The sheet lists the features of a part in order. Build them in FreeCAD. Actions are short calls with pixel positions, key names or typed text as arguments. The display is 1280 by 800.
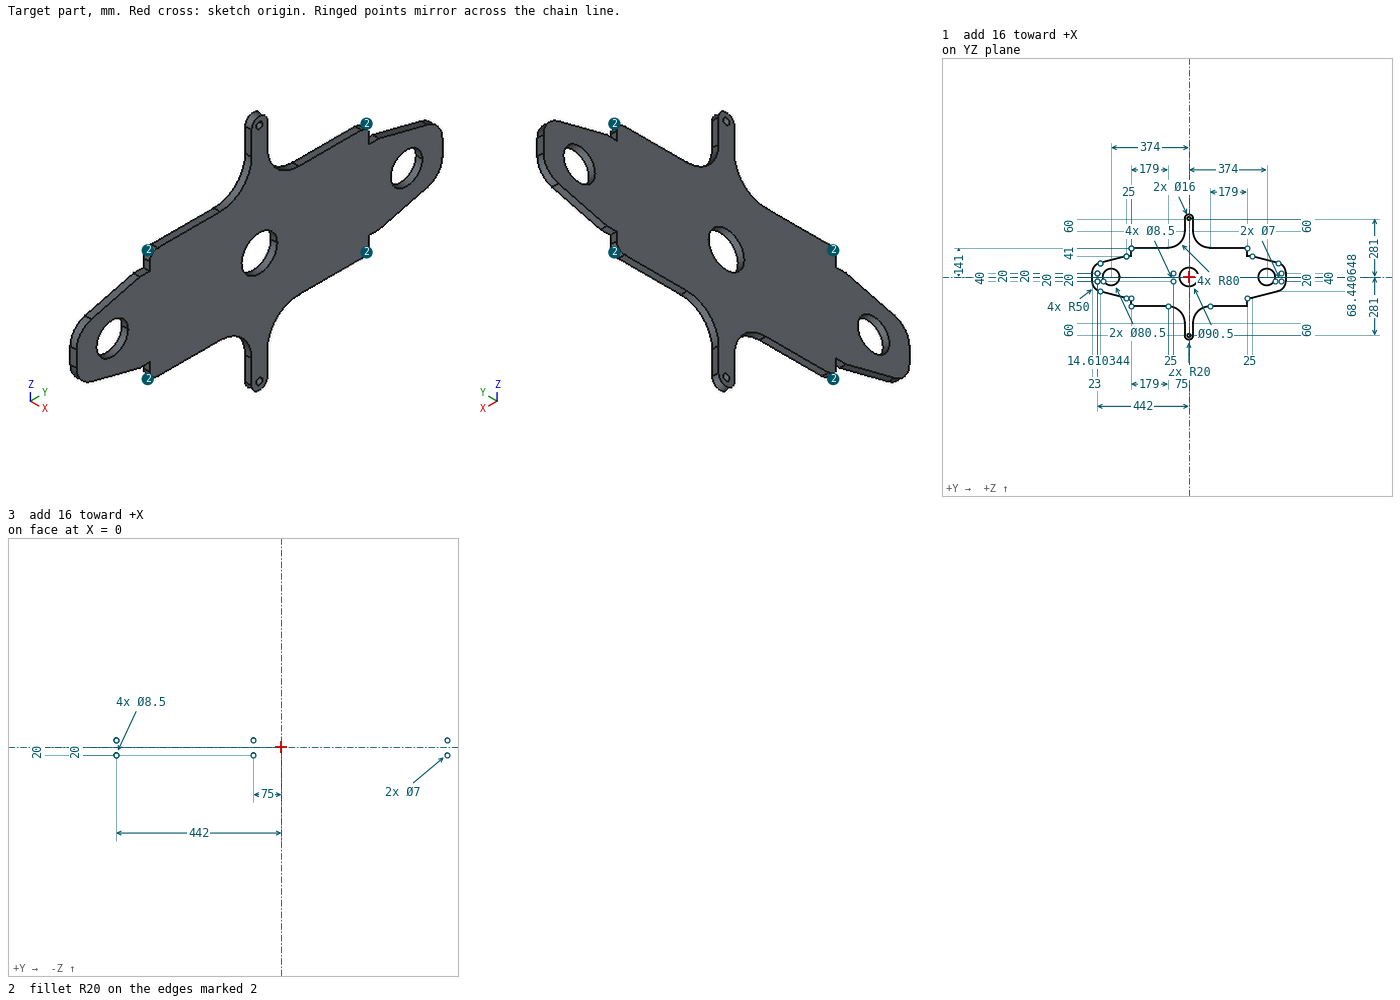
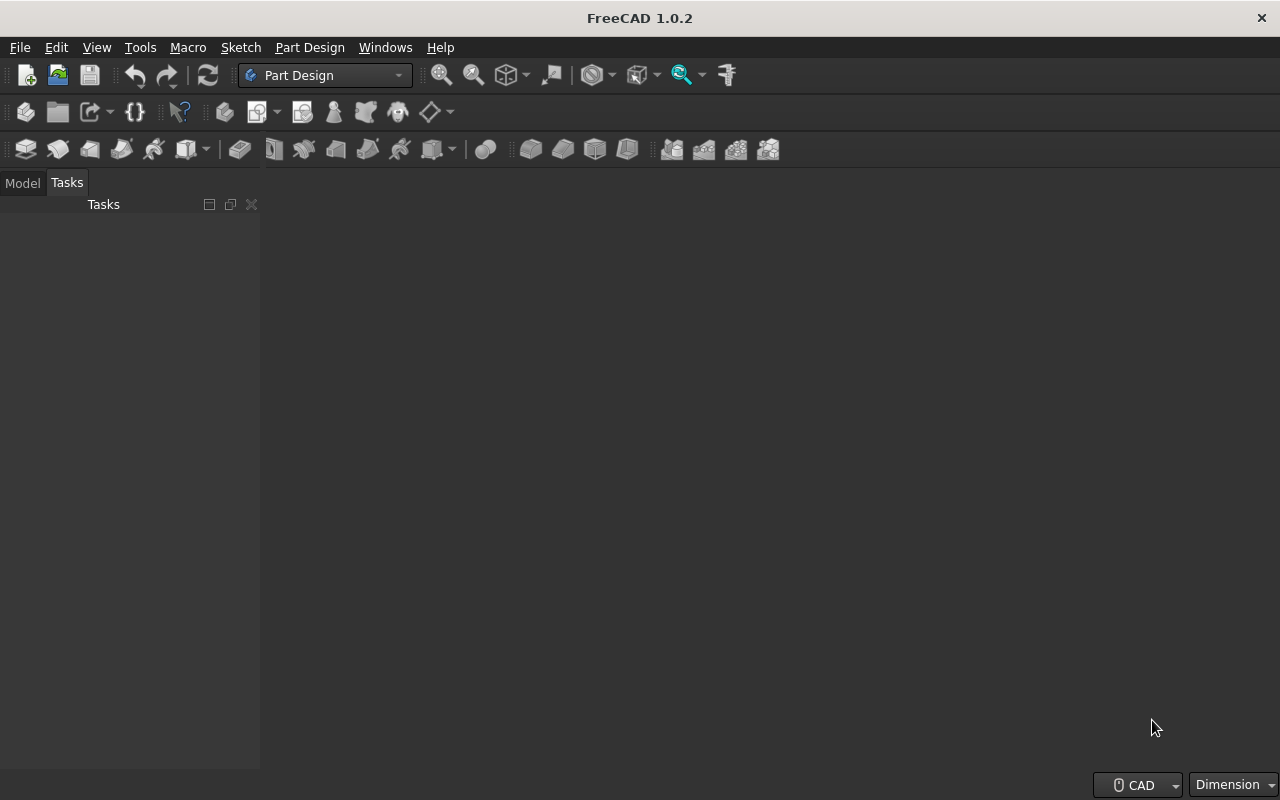
click(26, 76)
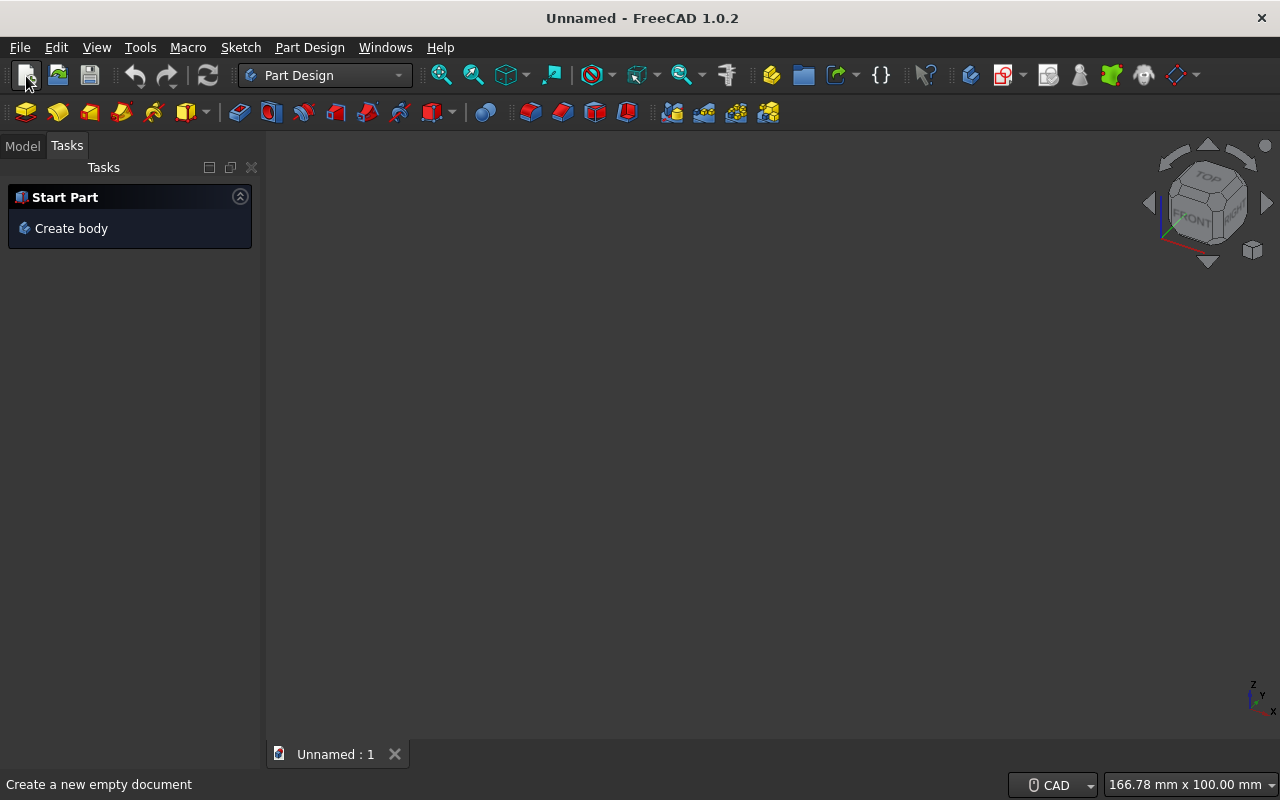
click(1004, 76)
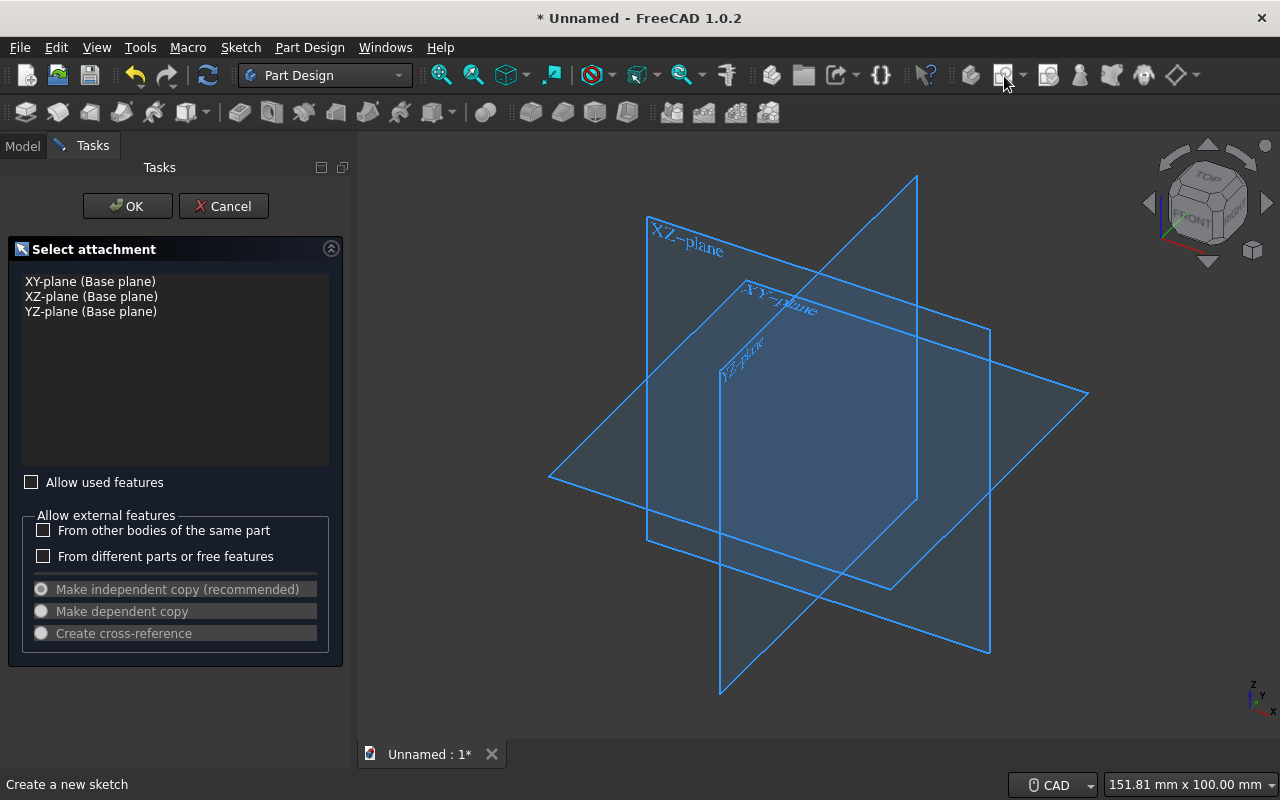
click(82, 312)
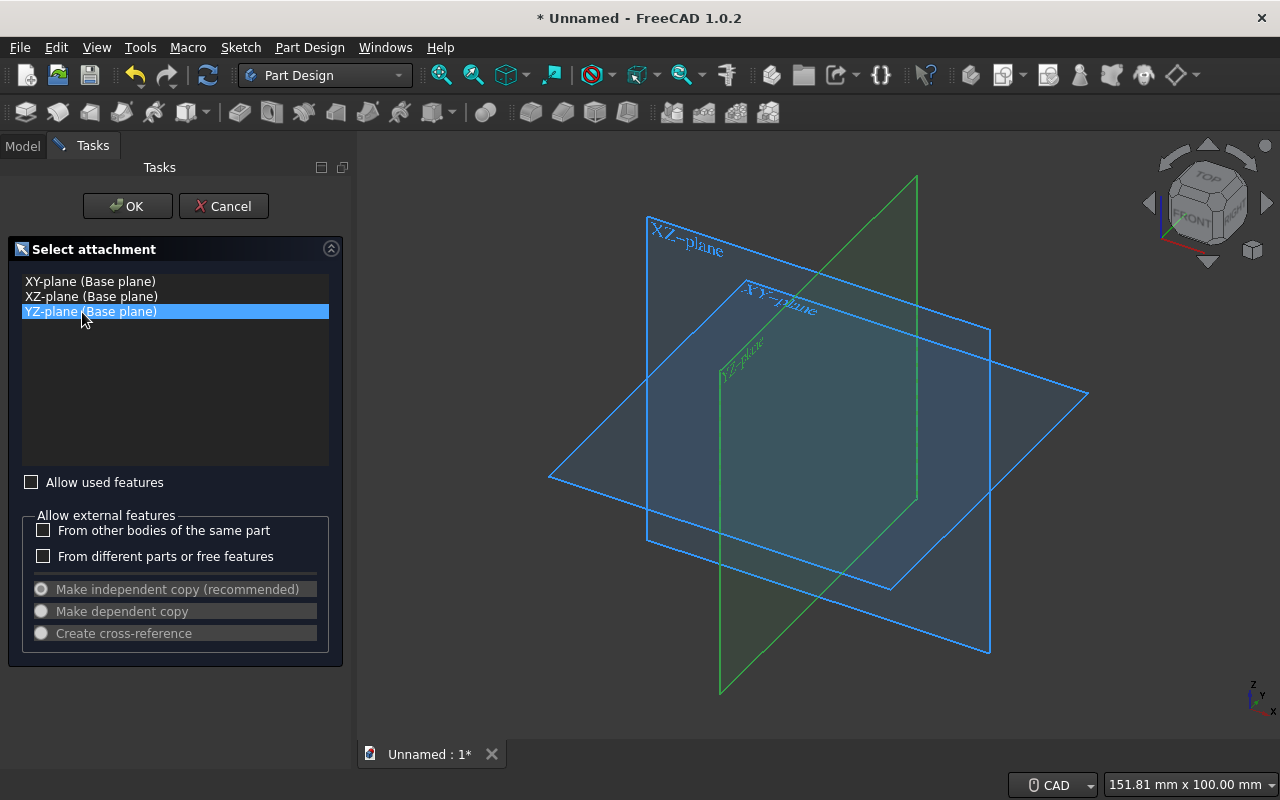
click(128, 206)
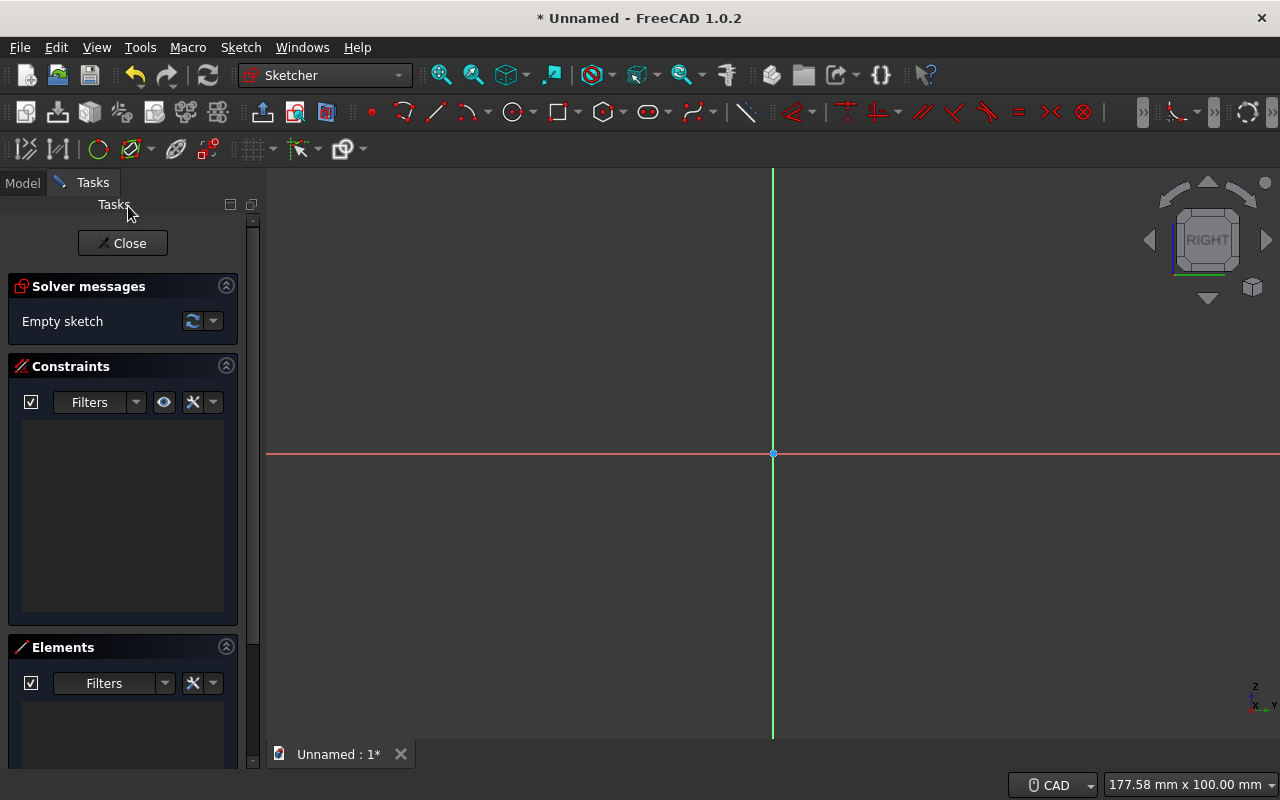
scroll(696, 454, down, 11)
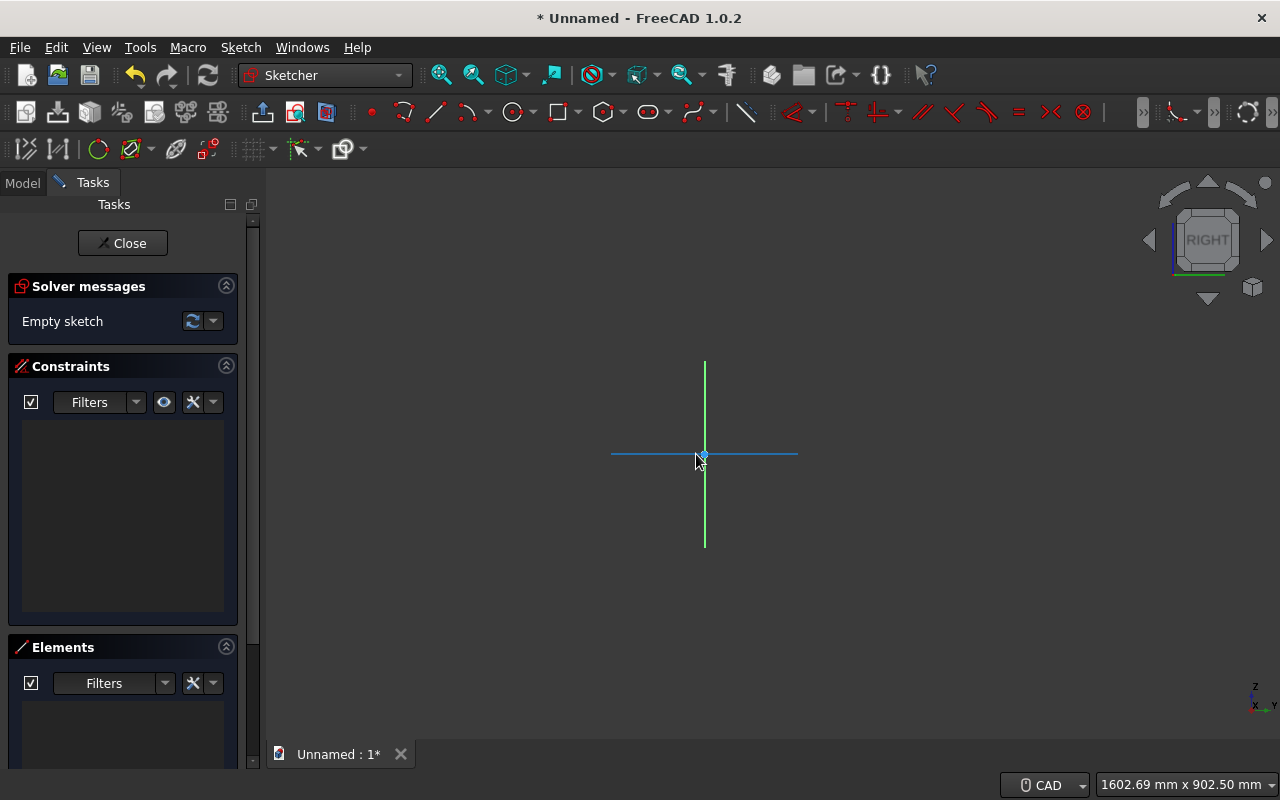
click(436, 112)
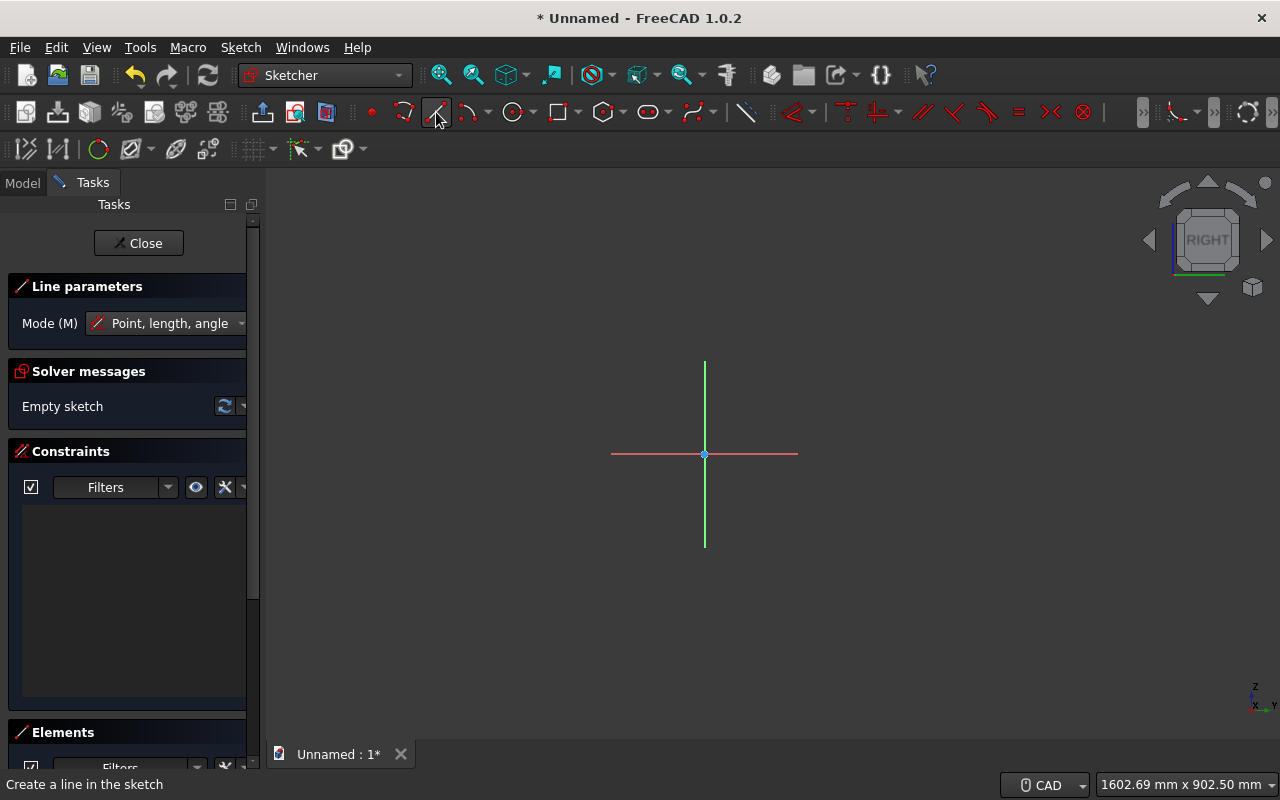
scroll(718, 315, up, 2)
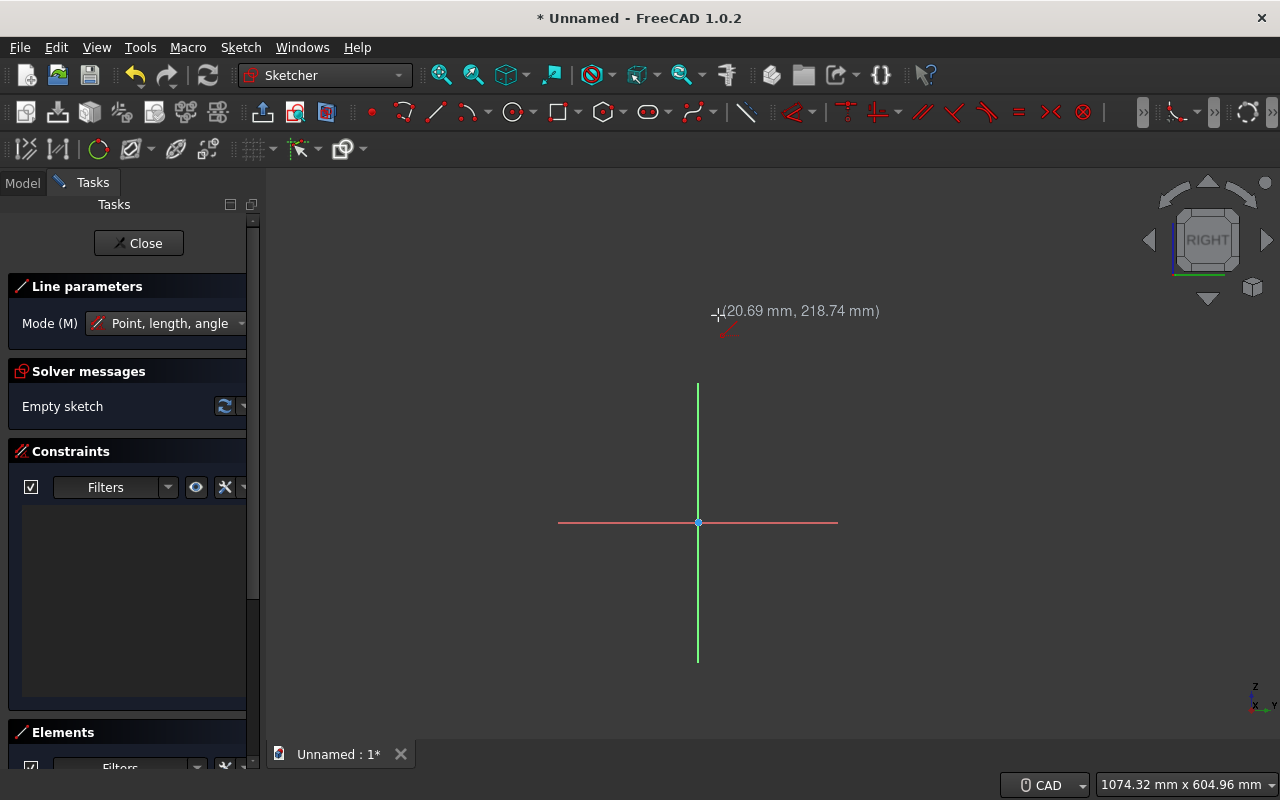
click(717, 314)
click(717, 258)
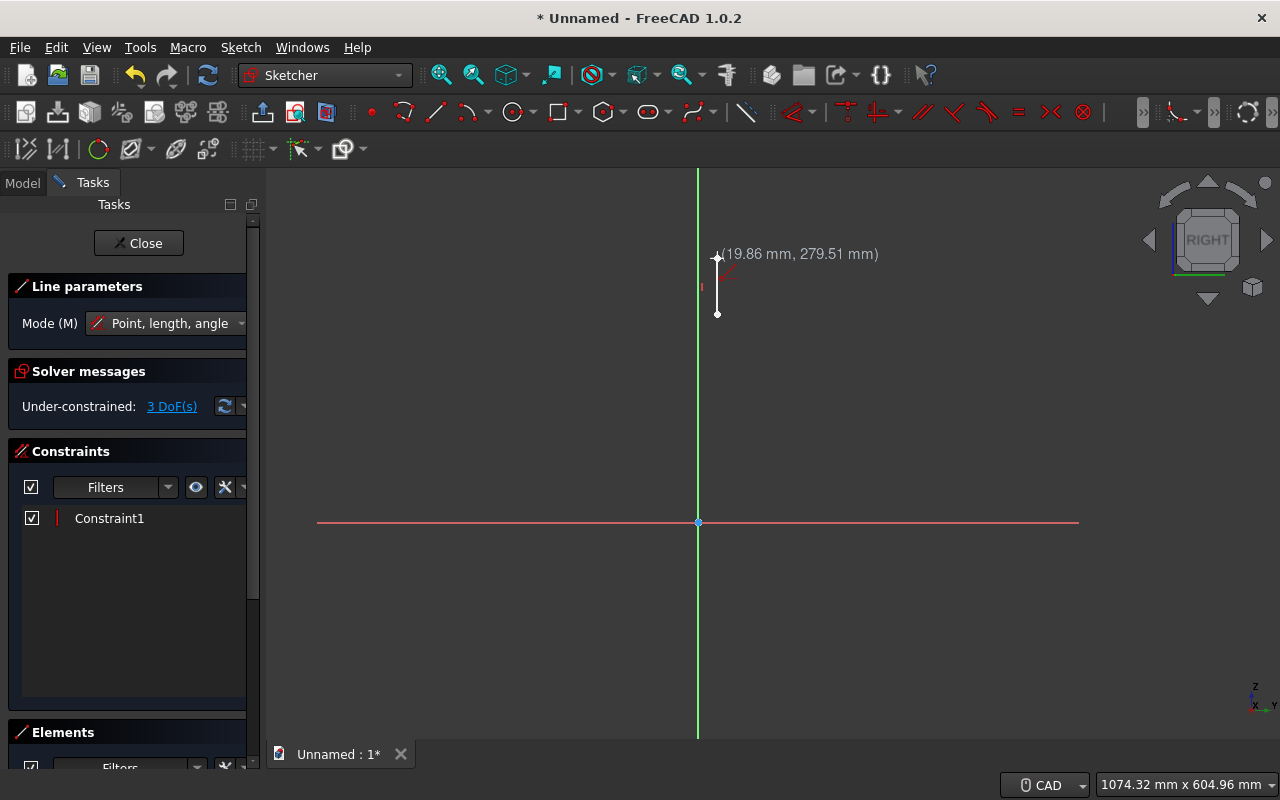
click(679, 258)
click(679, 314)